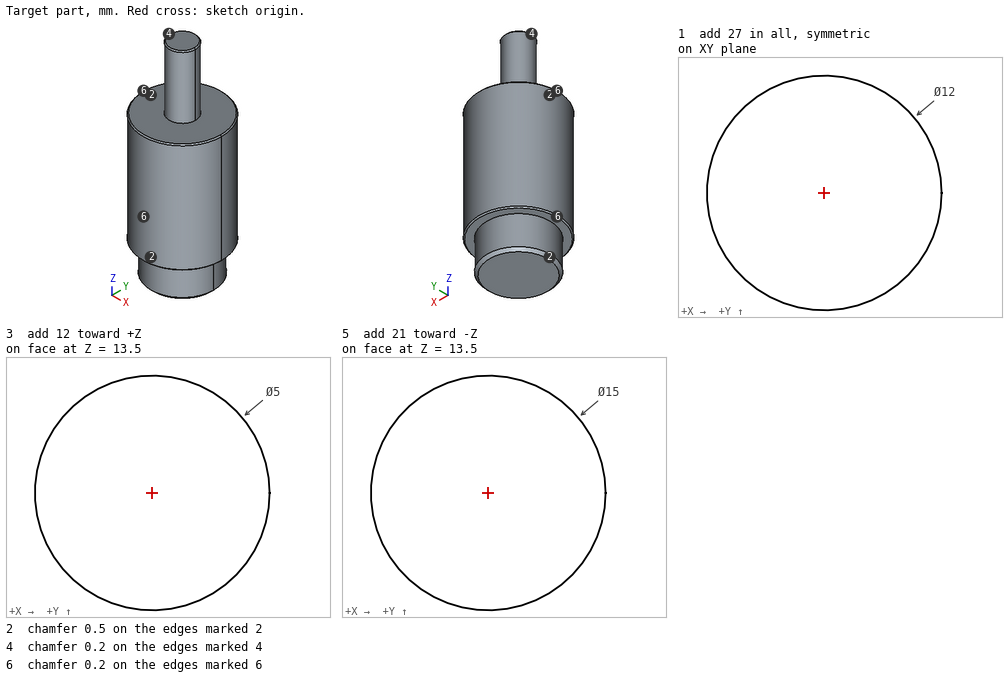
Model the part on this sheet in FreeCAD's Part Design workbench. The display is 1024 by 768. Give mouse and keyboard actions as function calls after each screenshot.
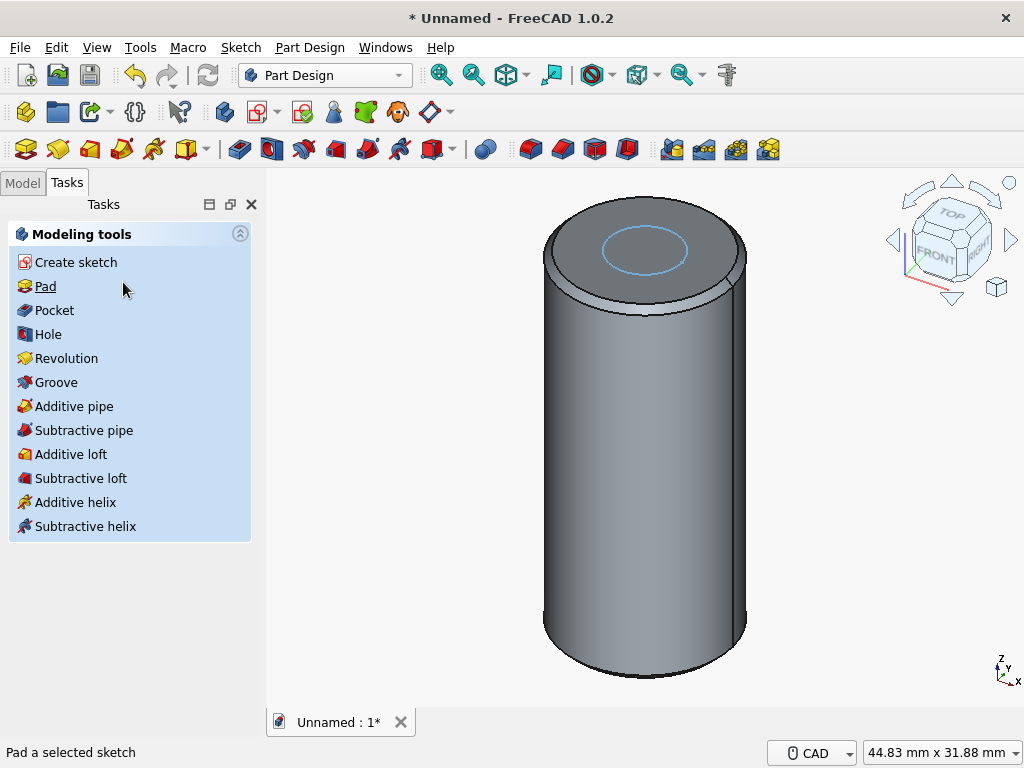
click(26, 150)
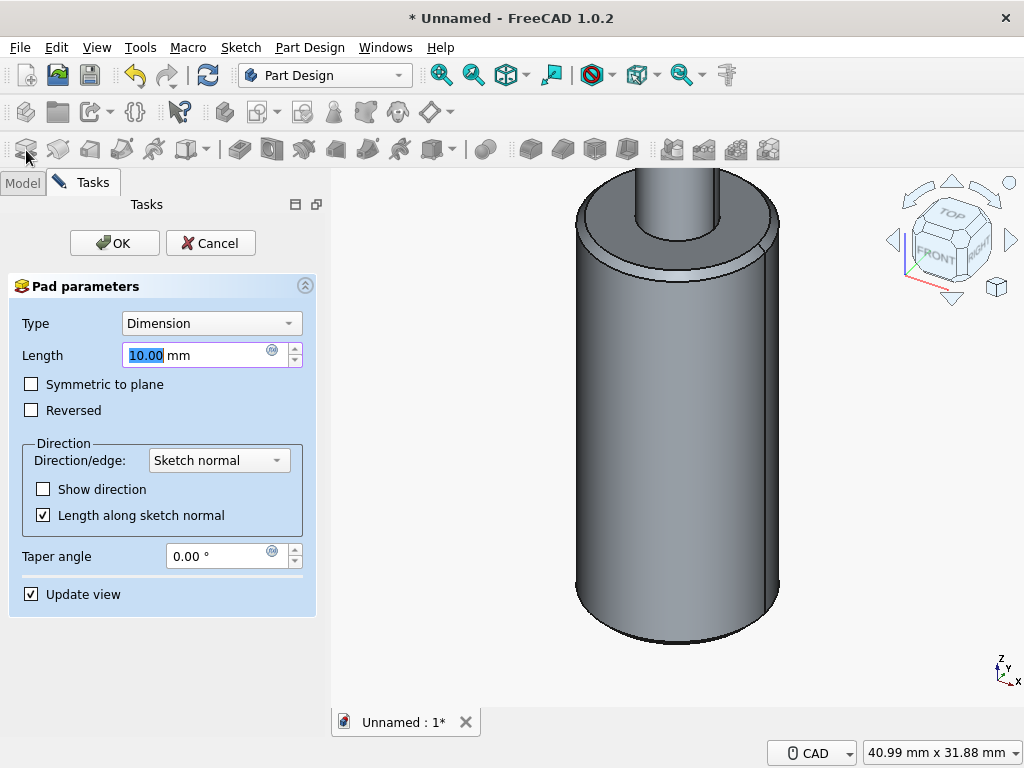
text(12)
key(Tab)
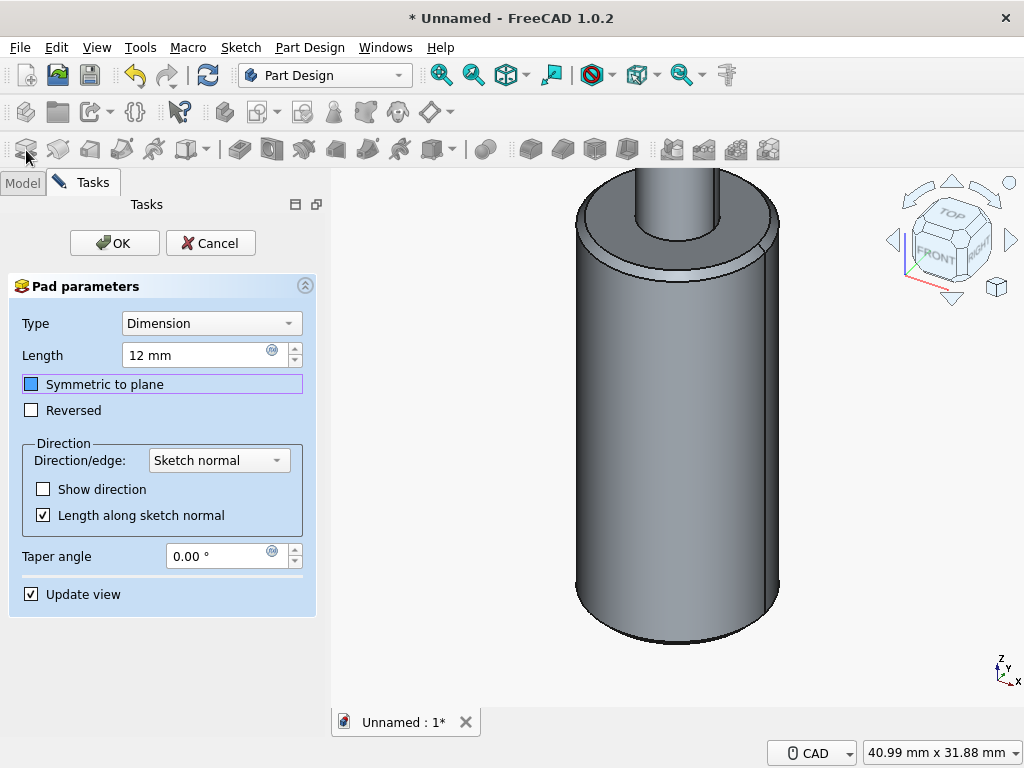
click(115, 243)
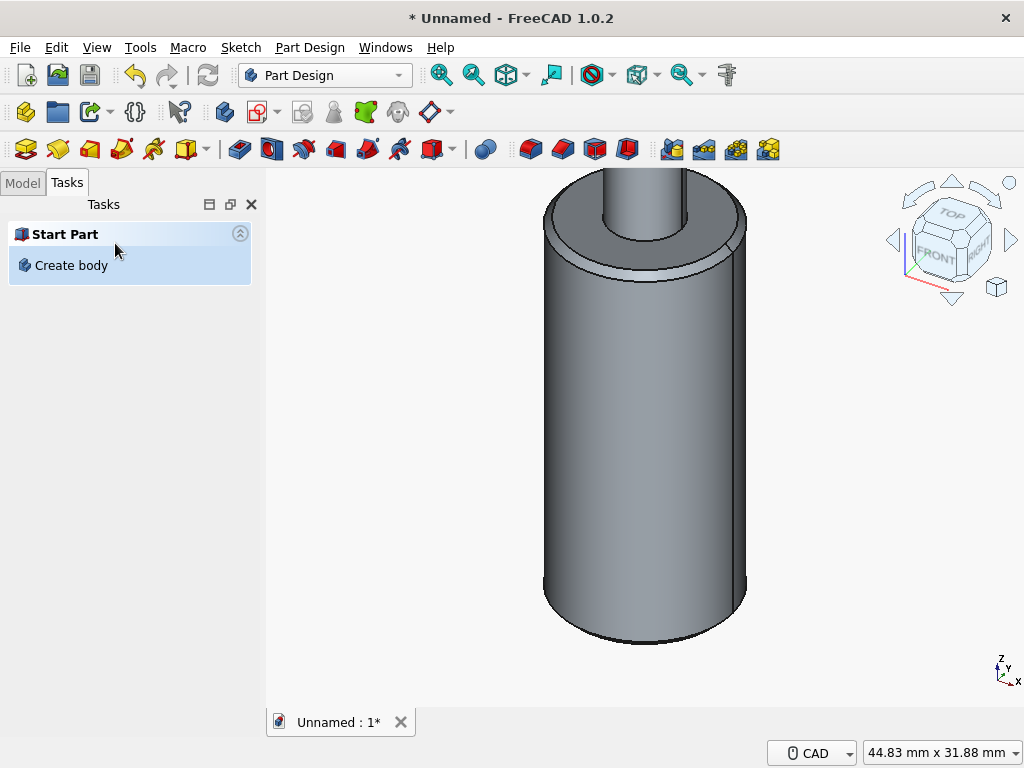
click(442, 76)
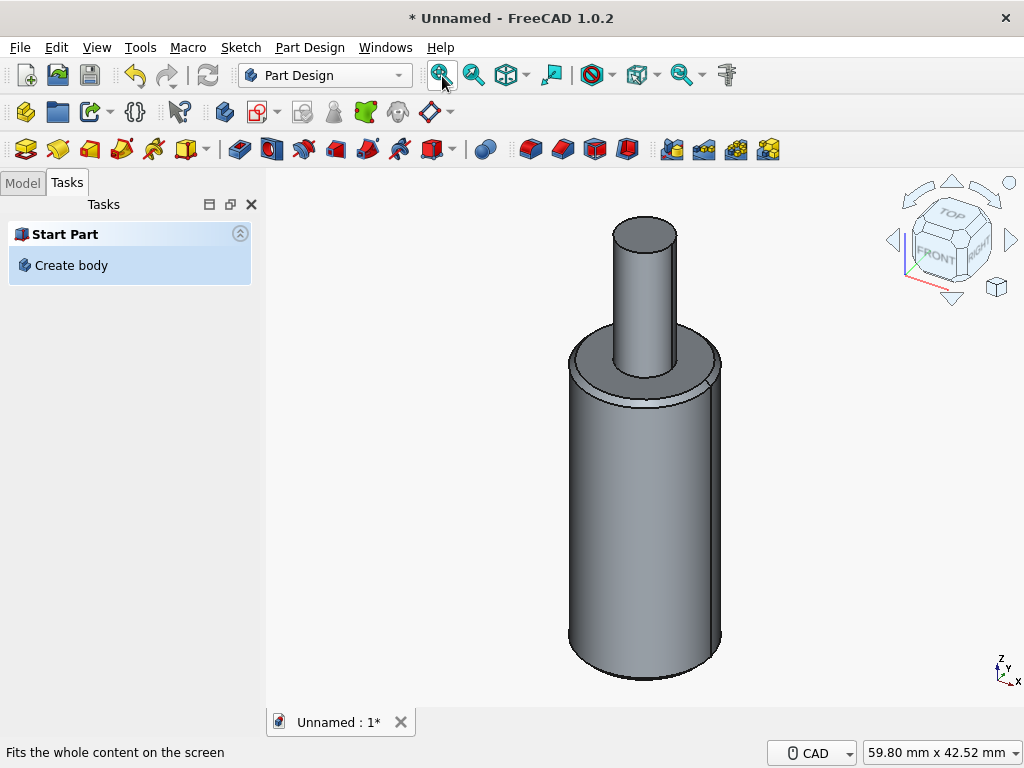
click(613, 236)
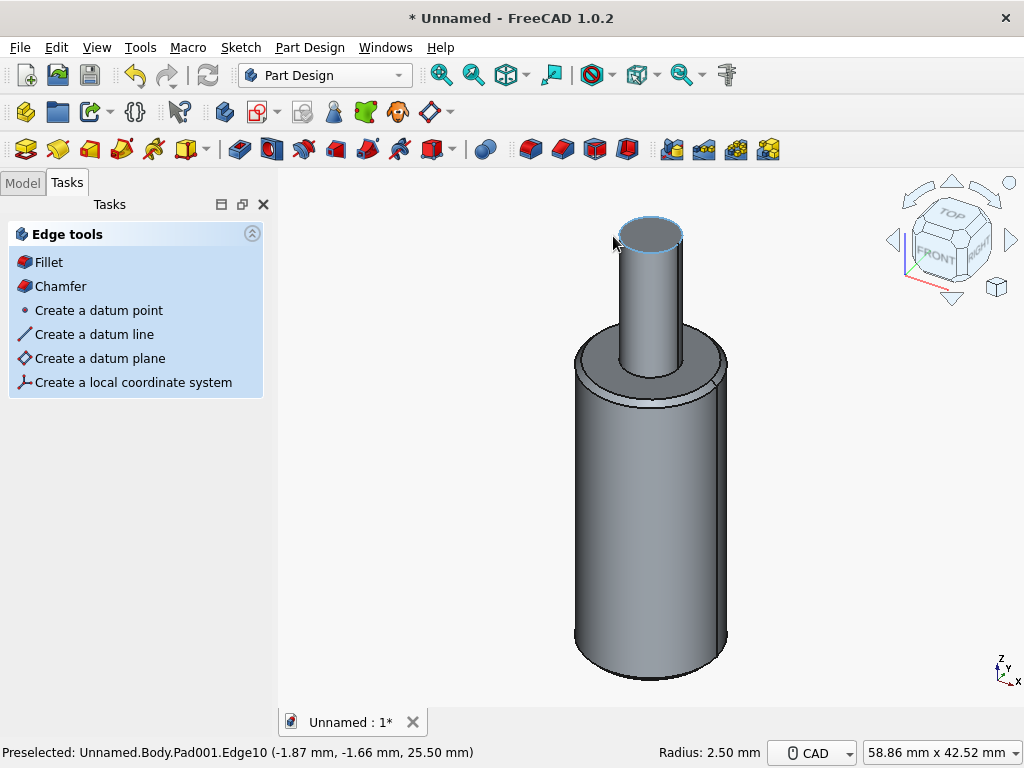
click(564, 150)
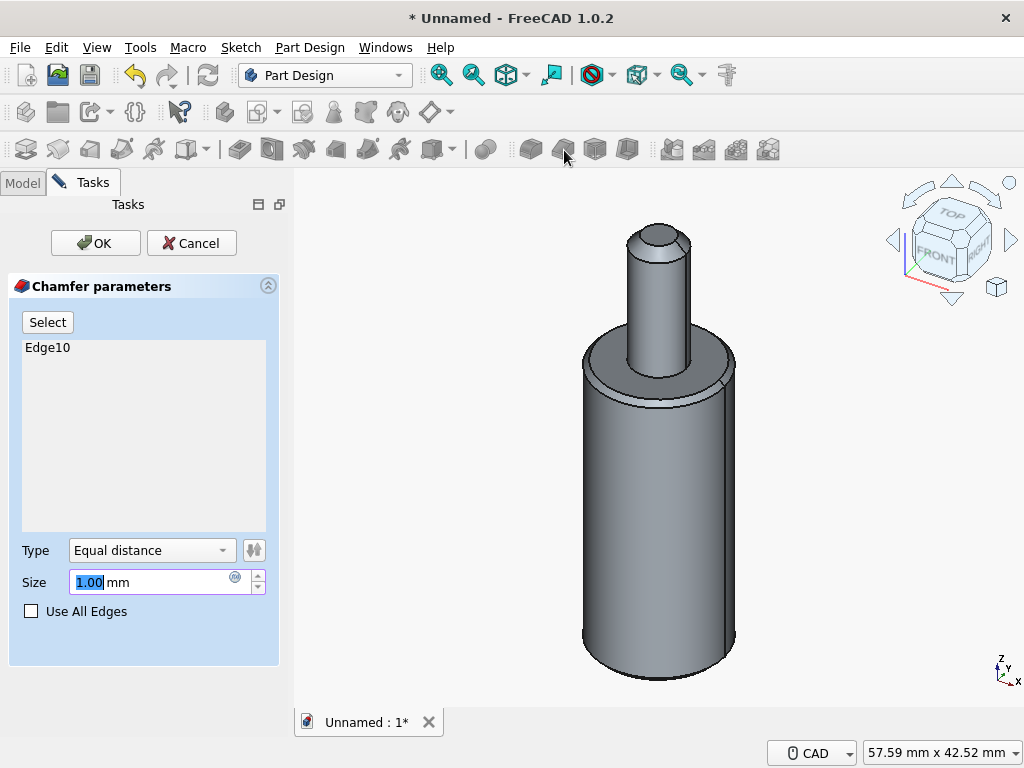
text(0.2)
key(Tab)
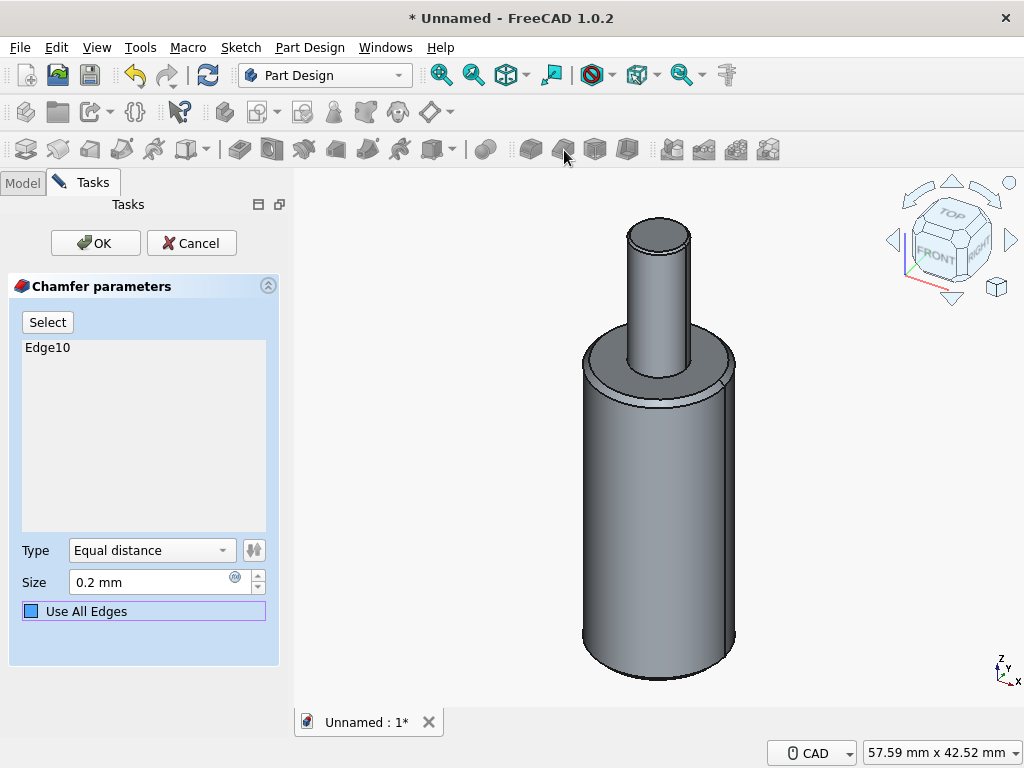
click(96, 243)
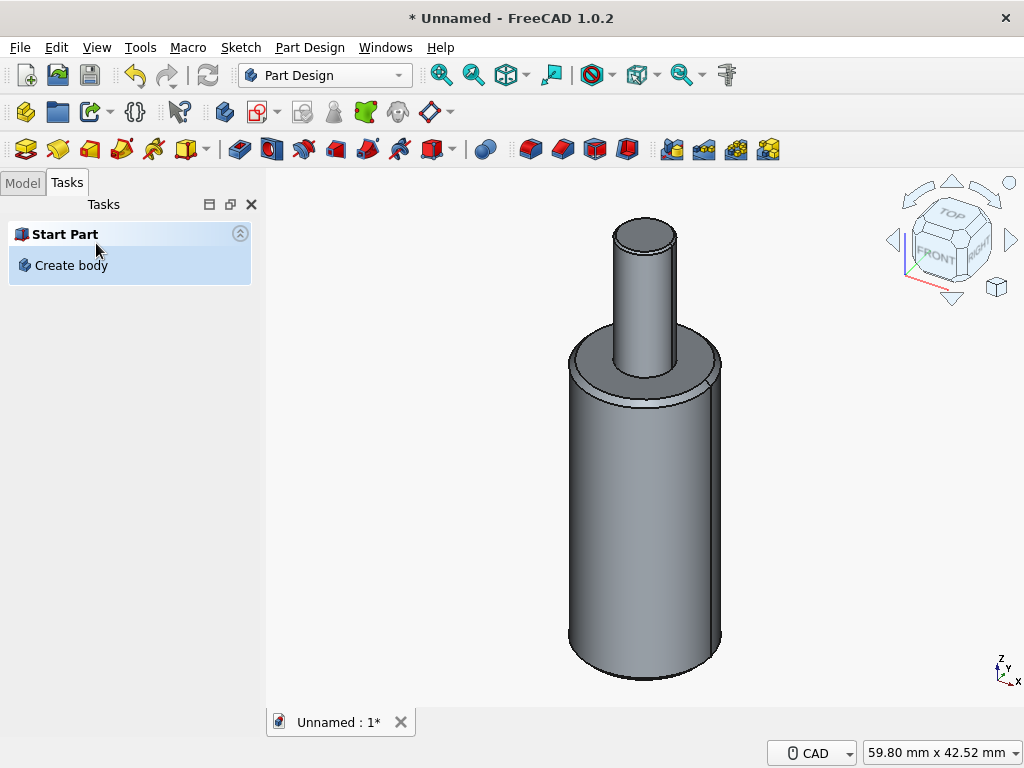
click(699, 350)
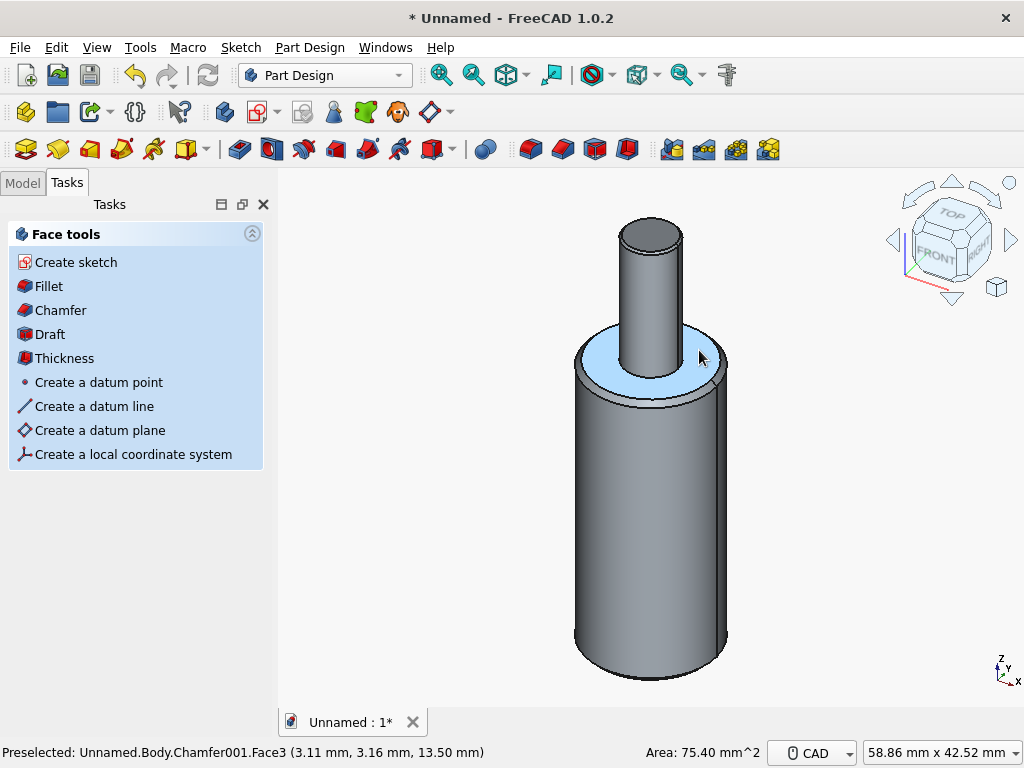
click(258, 112)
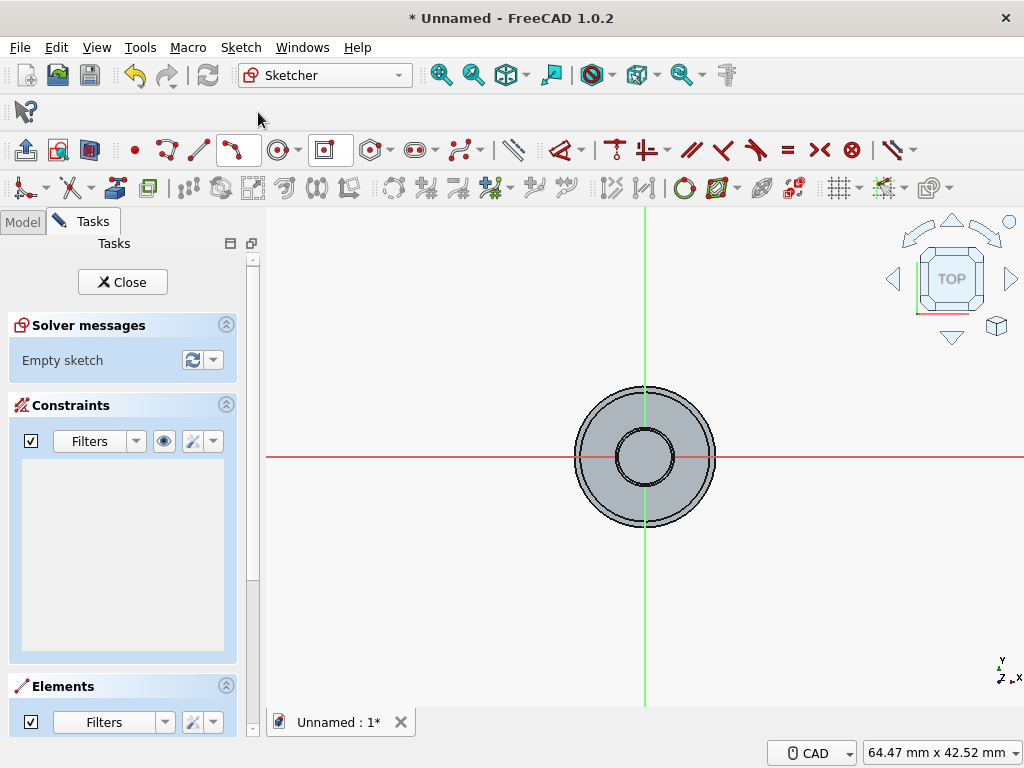
scroll(728, 457, up, 3)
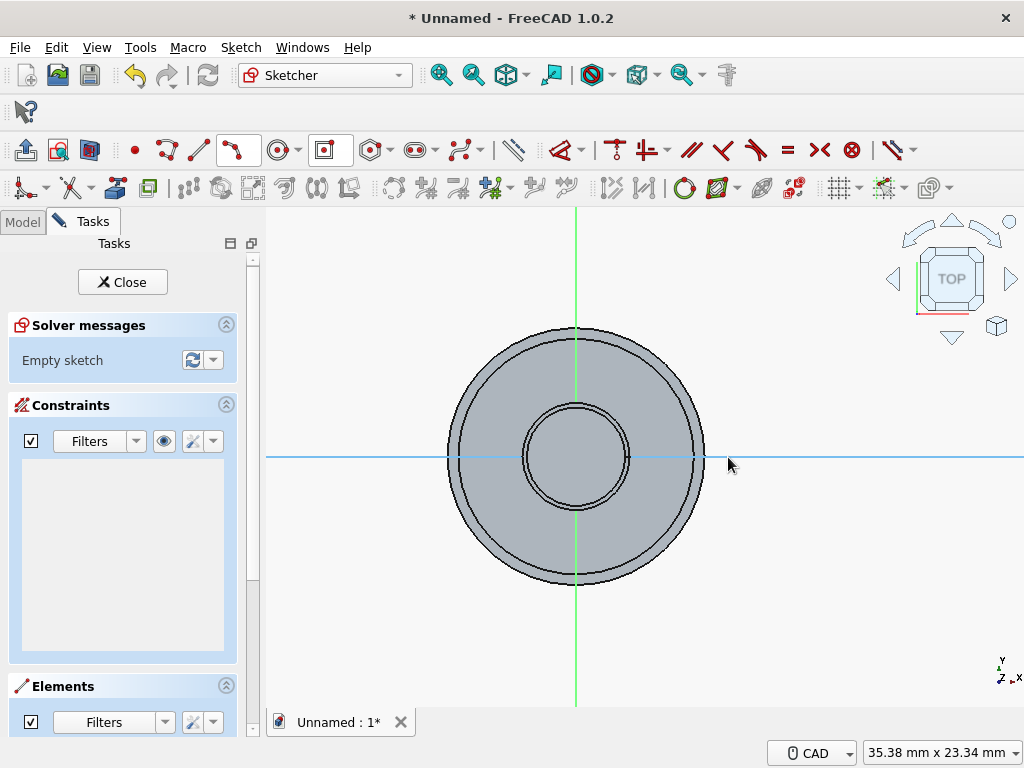
click(278, 150)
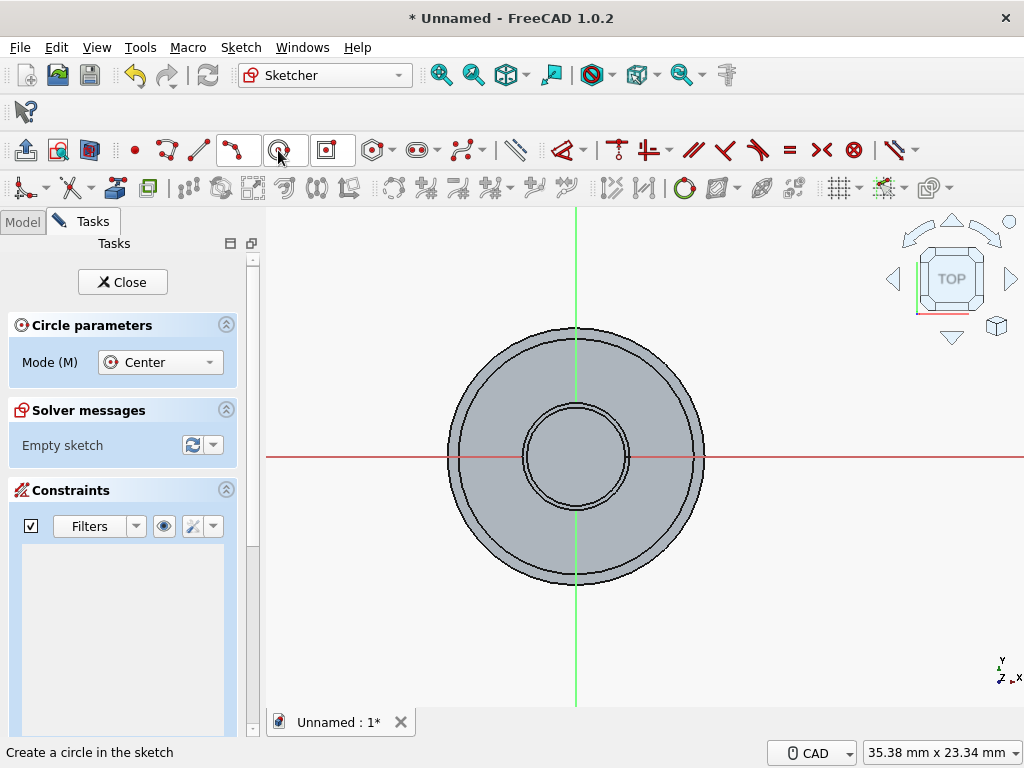
click(576, 457)
move(690, 343)